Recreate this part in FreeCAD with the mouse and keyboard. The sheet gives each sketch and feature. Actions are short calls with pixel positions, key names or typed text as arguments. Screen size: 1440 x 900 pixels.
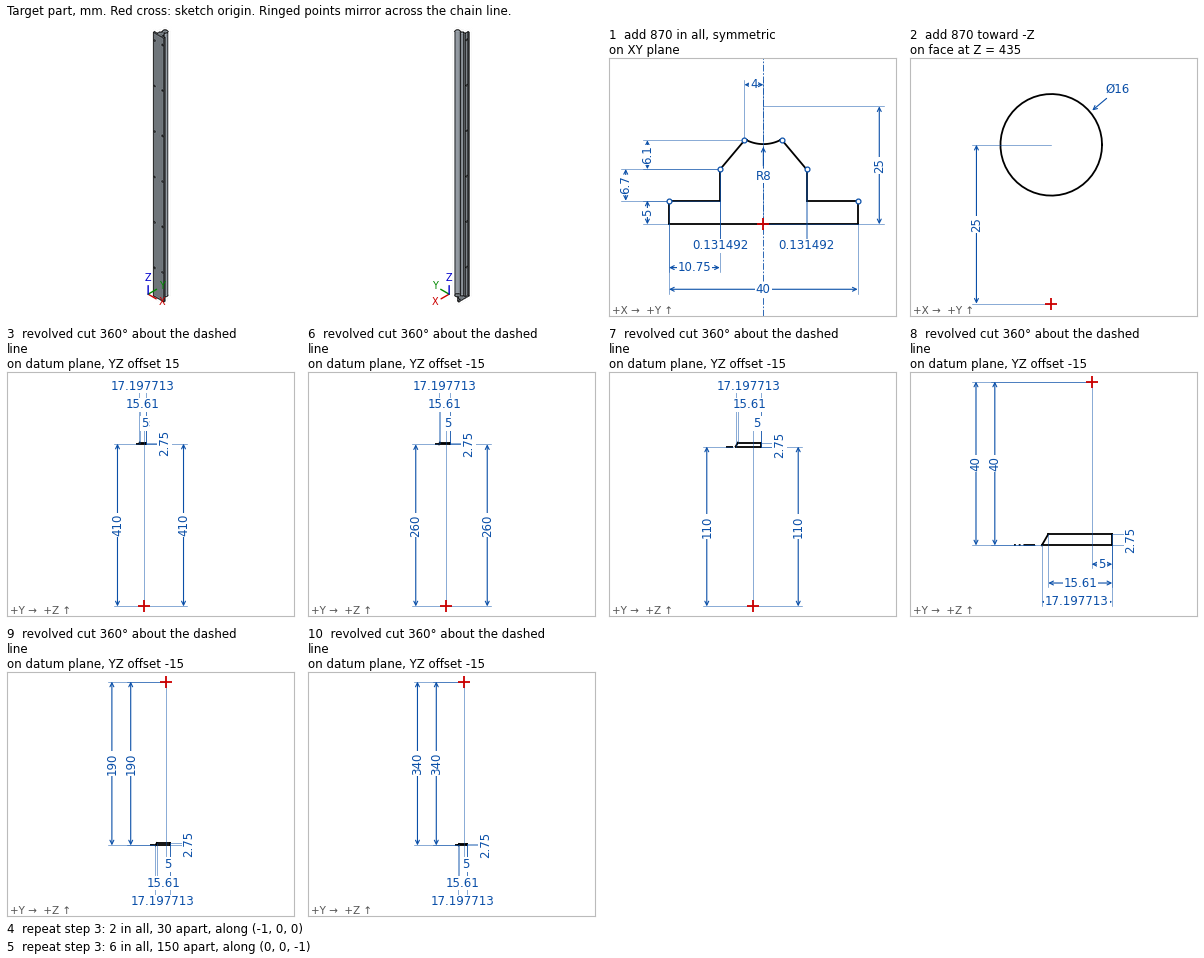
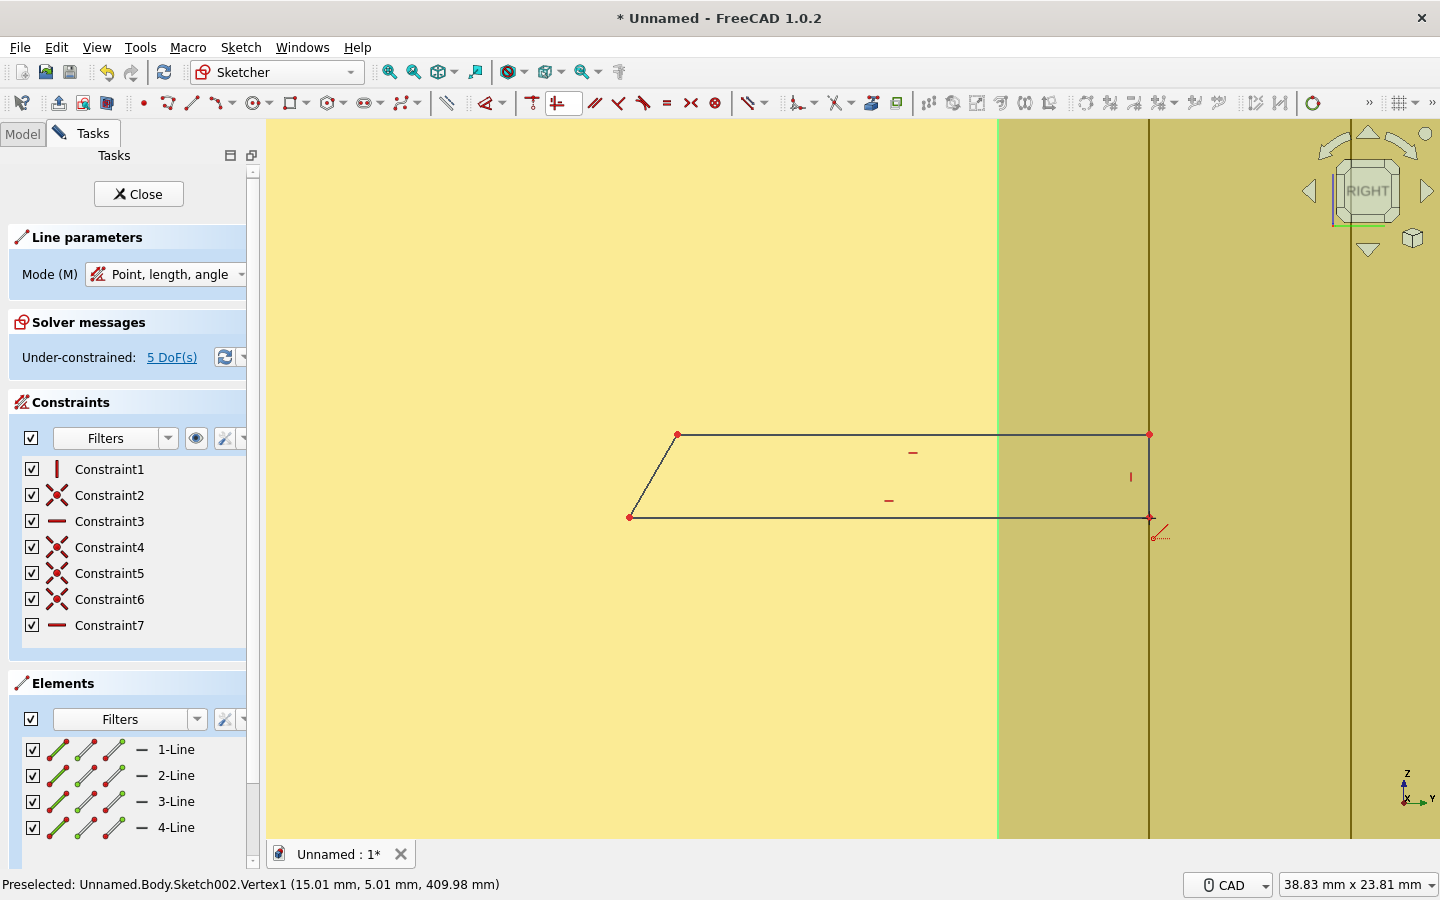
click(577, 517)
click(421, 517)
key(Escape)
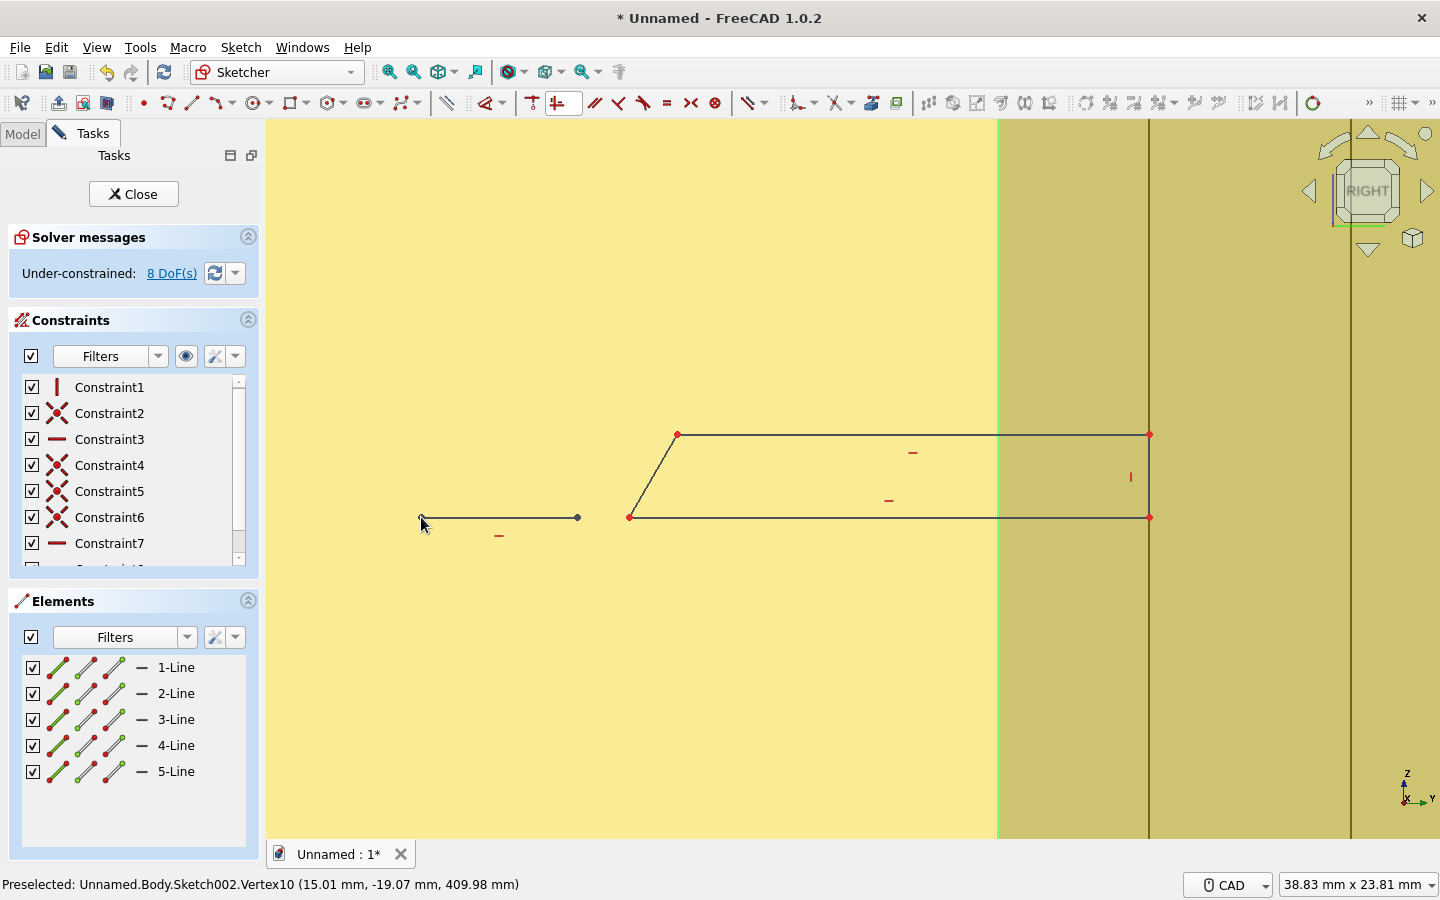
click(530, 518)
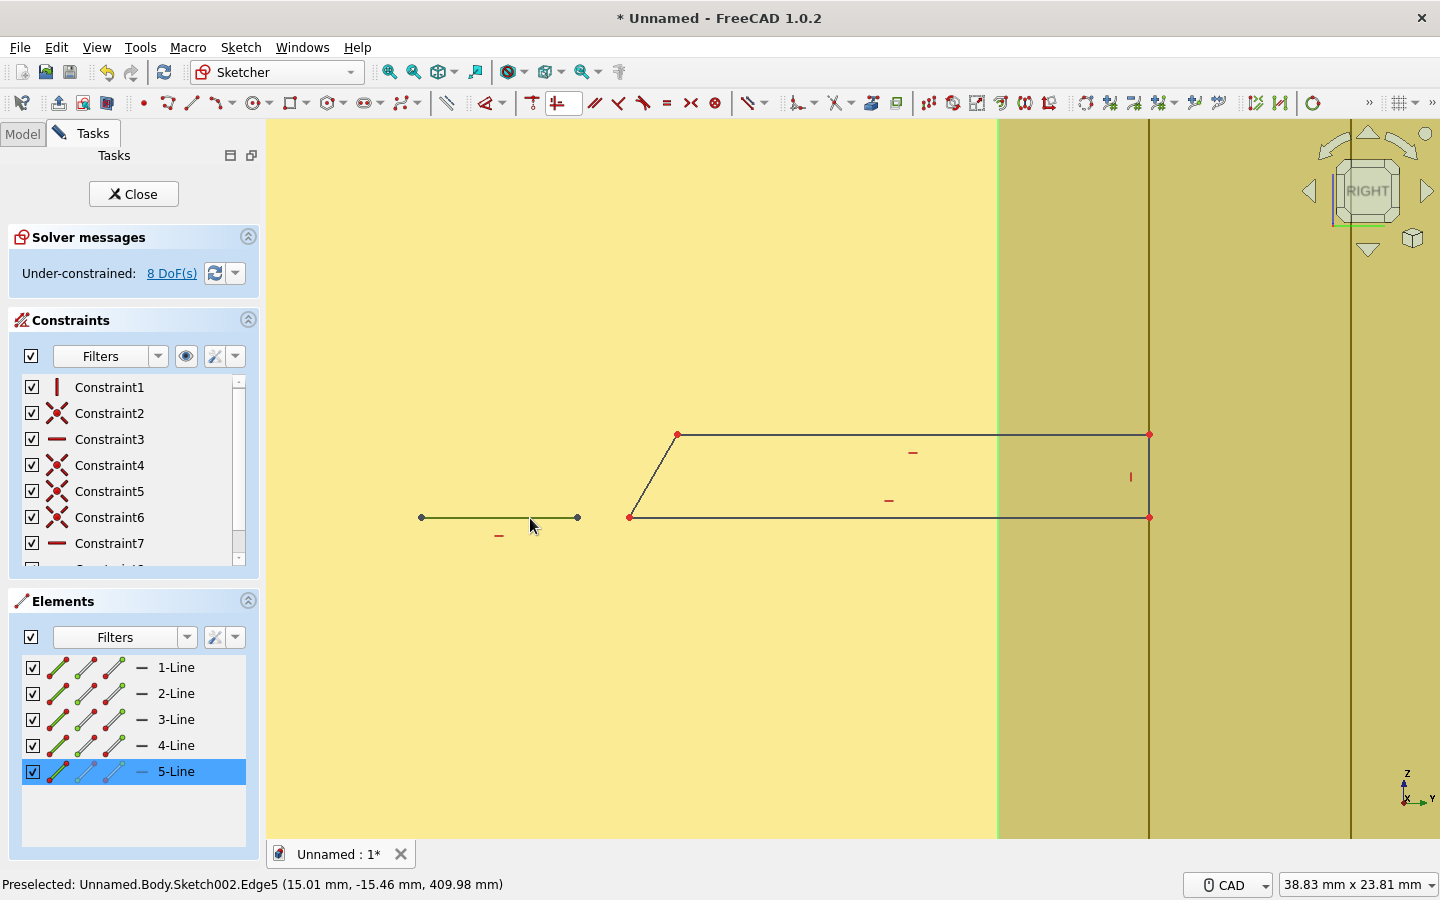
key(g)
key(n)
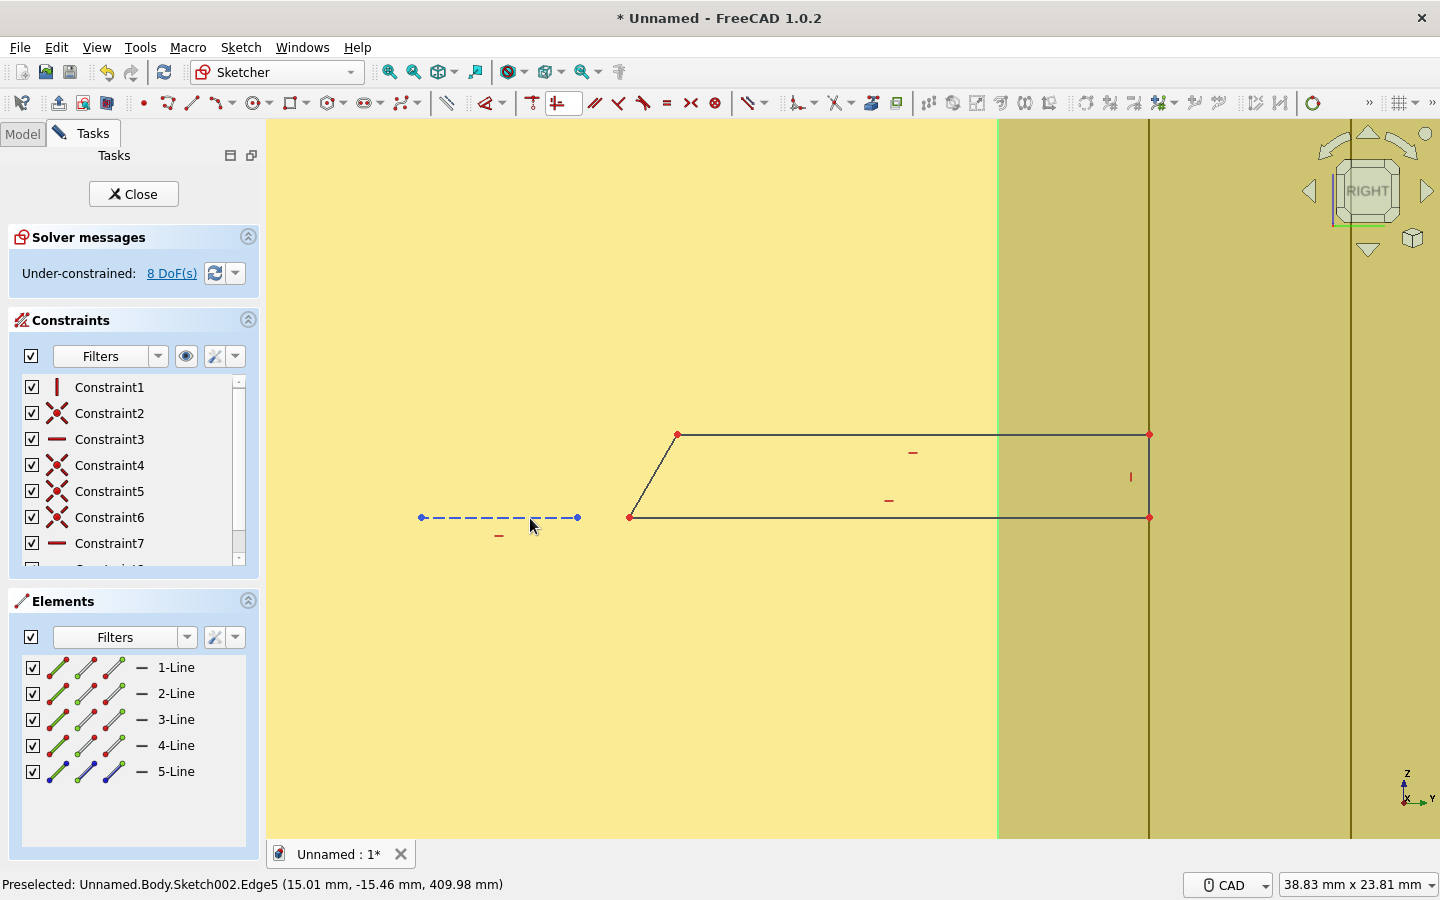
click(486, 104)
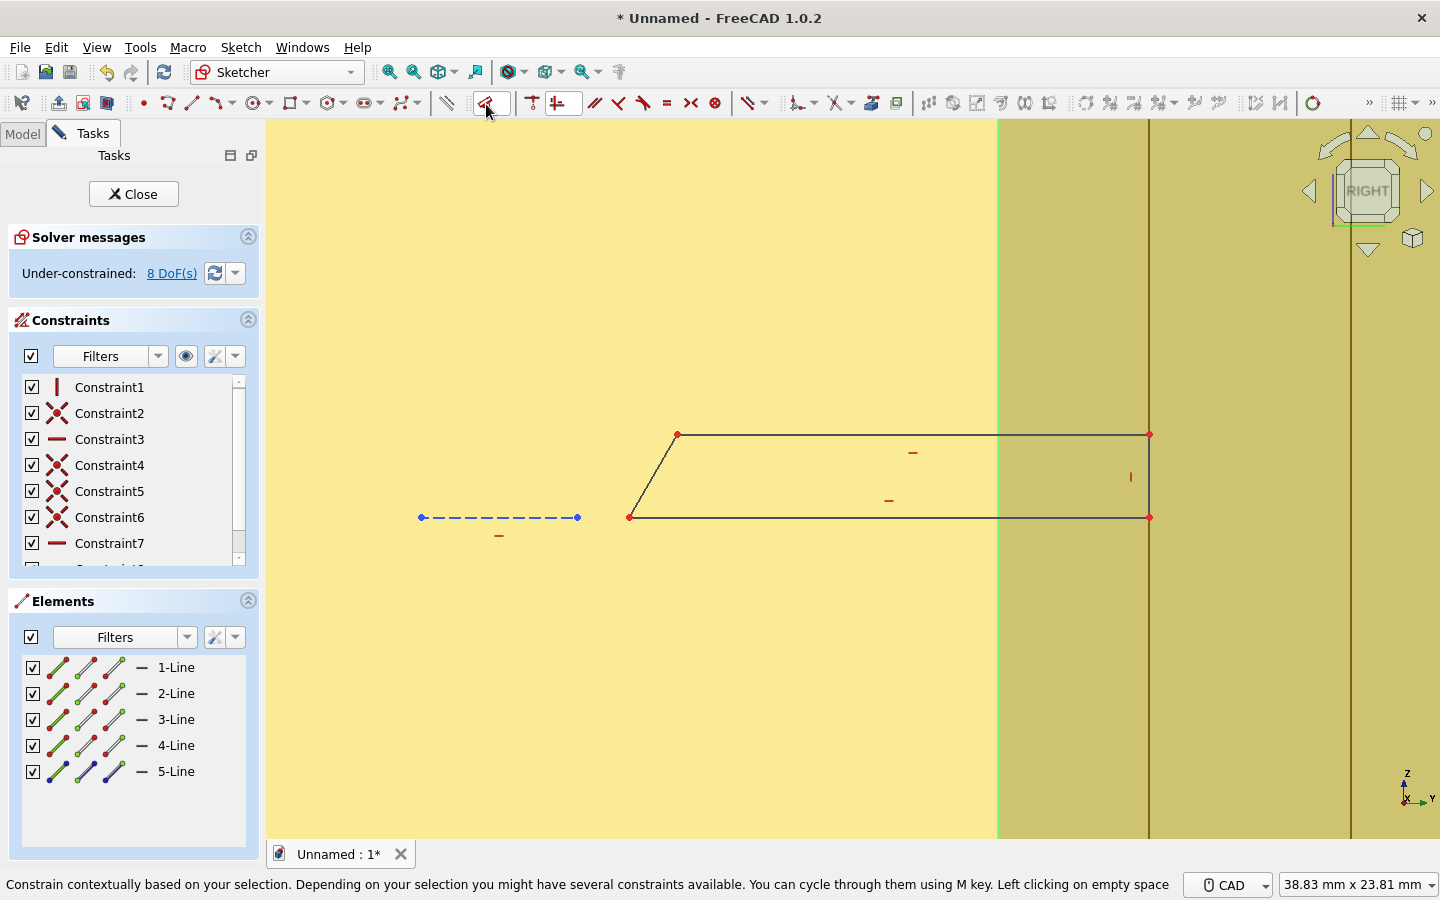
click(1149, 518)
click(1073, 484)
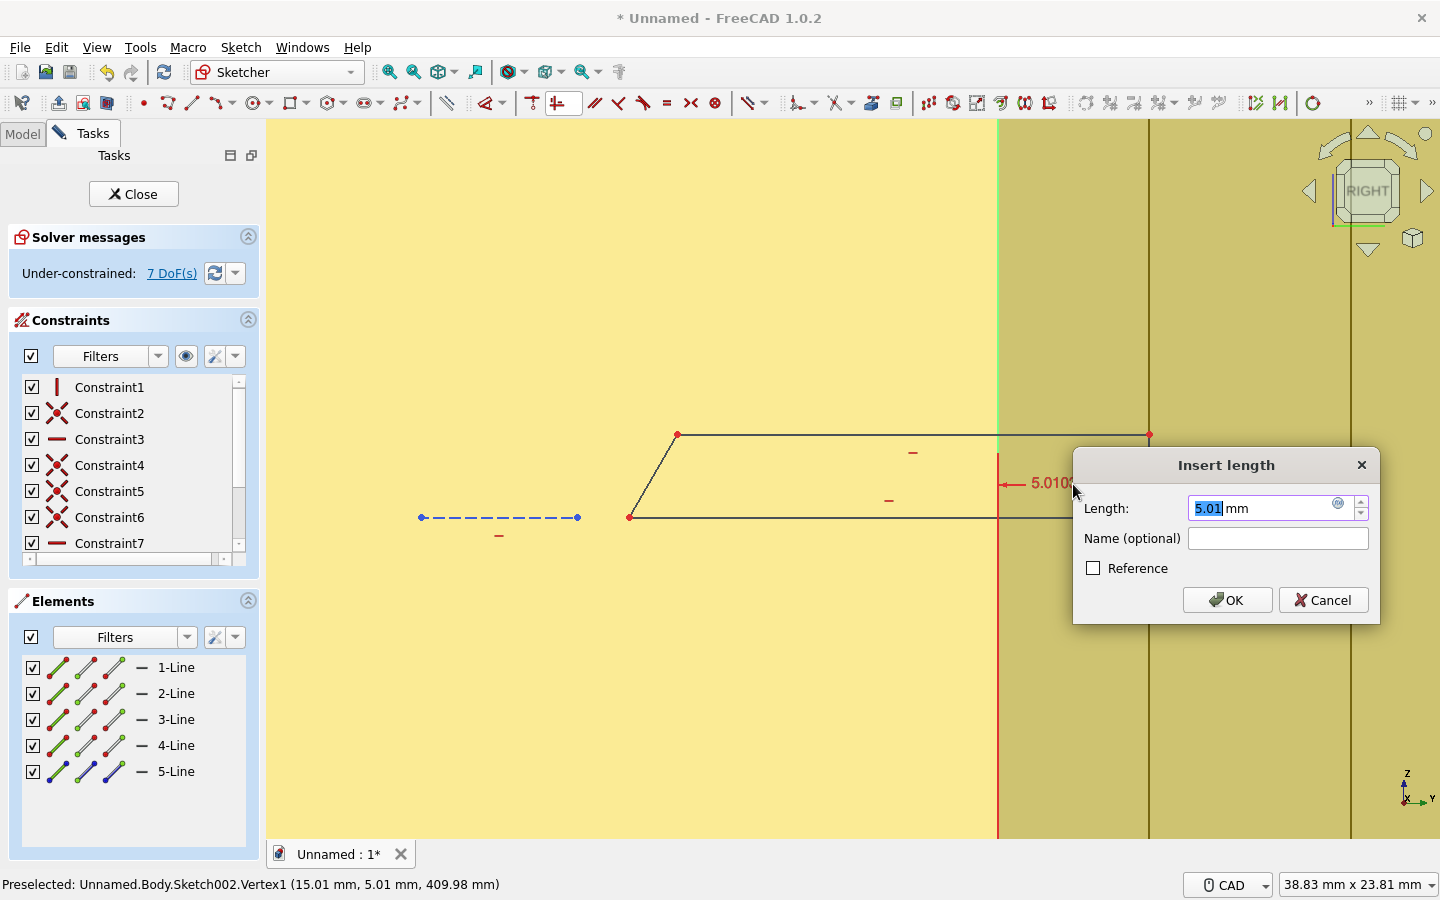
text(5)
key(Return)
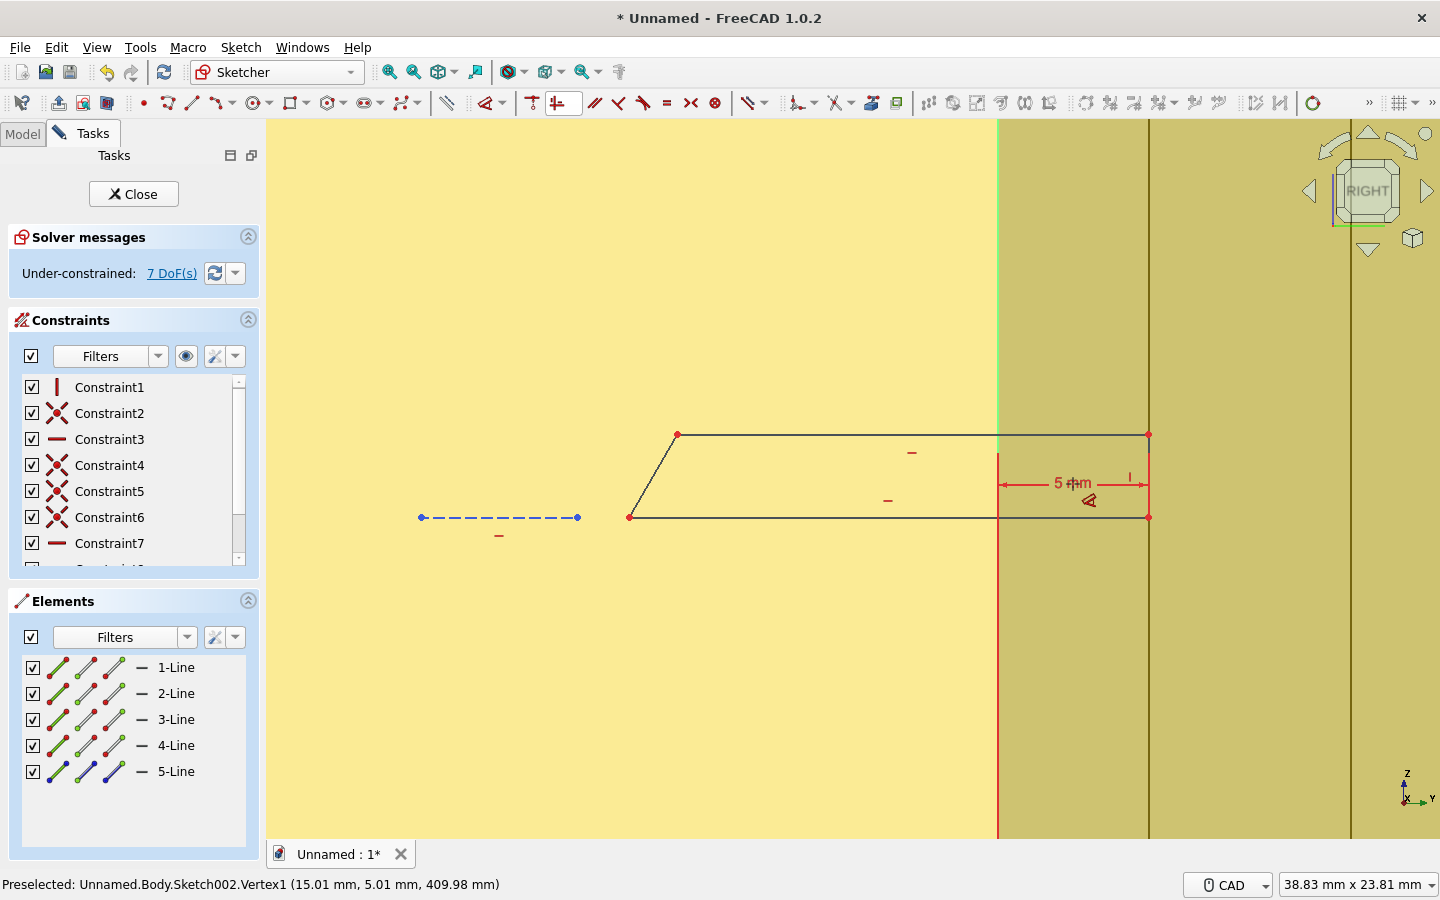
click(1149, 493)
click(1183, 476)